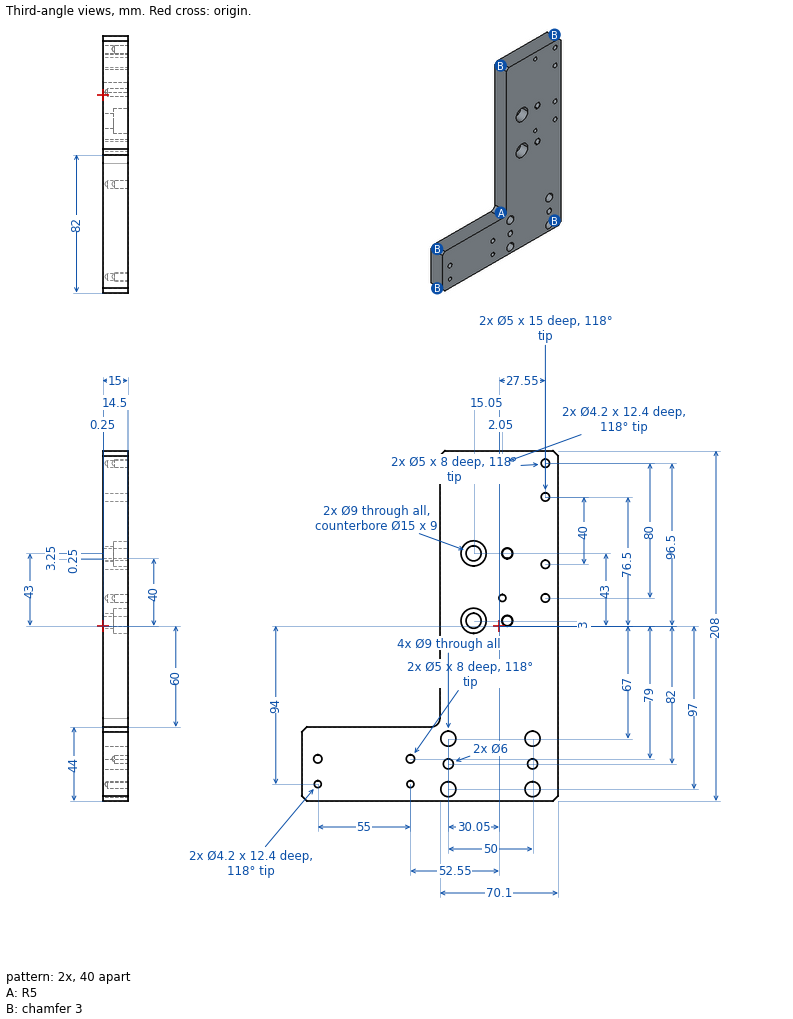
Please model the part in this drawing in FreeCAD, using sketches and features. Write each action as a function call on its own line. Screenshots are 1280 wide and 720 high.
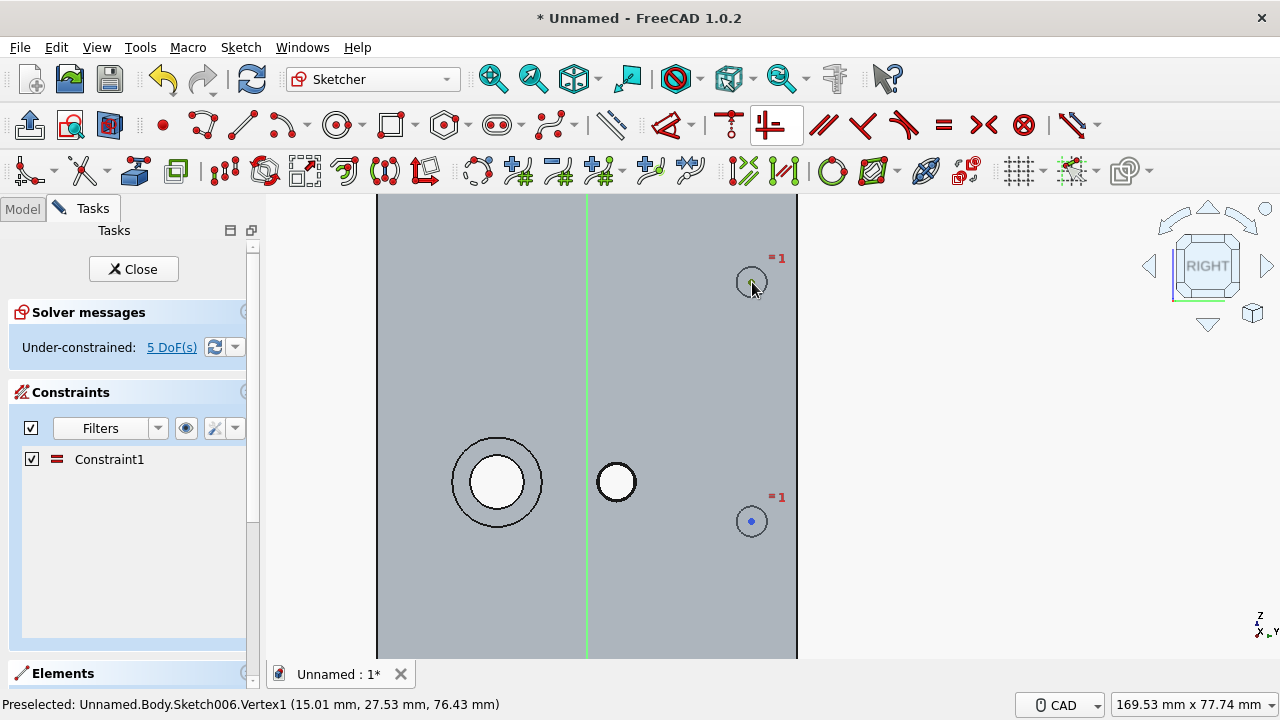
click(752, 521)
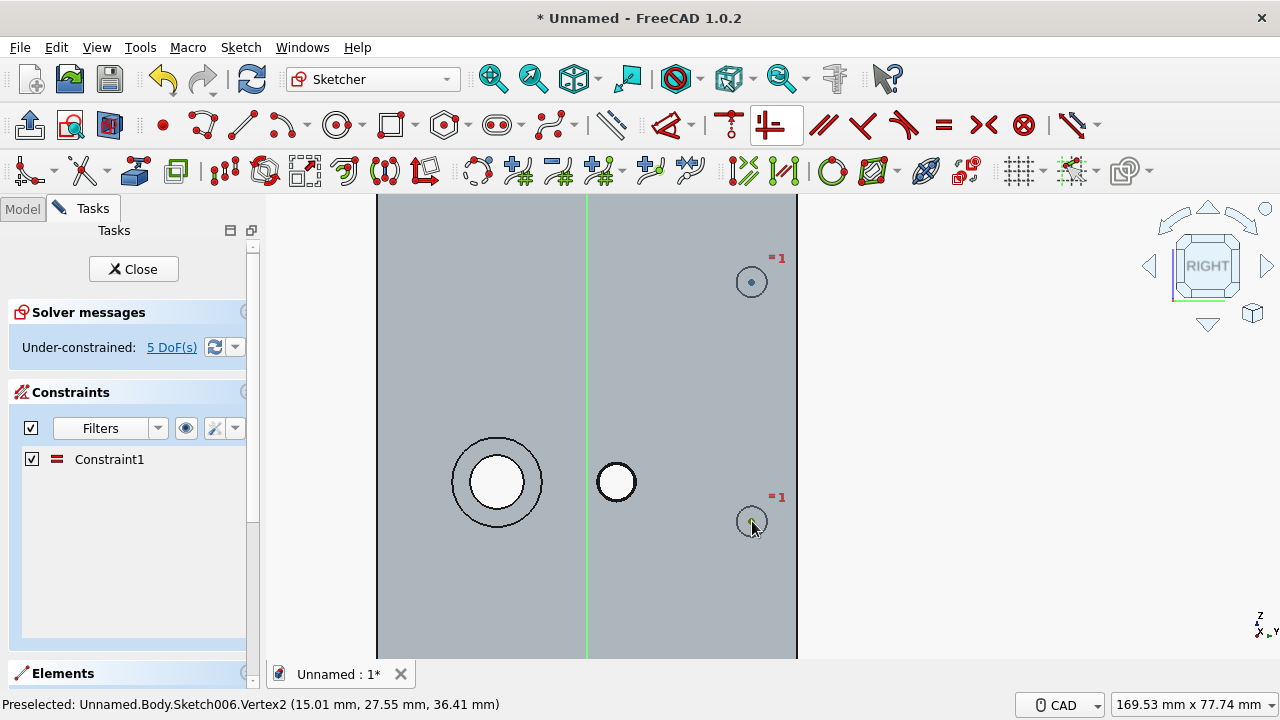
click(798, 126)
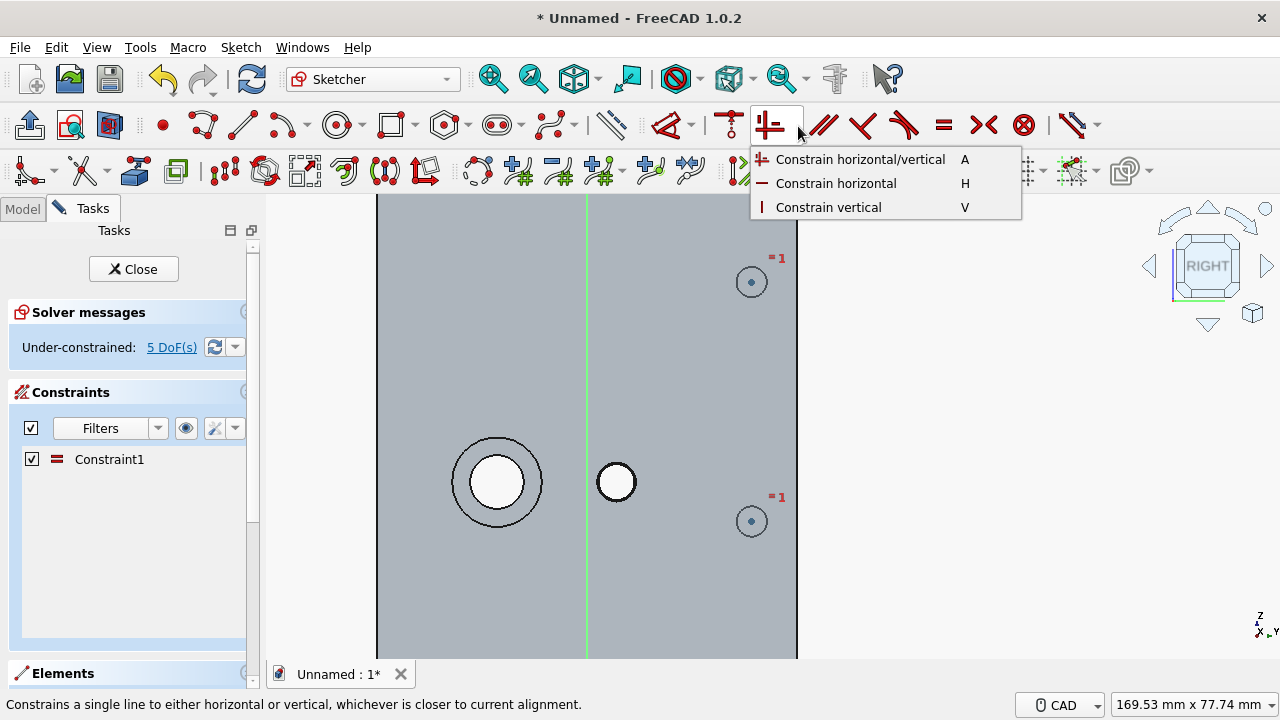
click(886, 207)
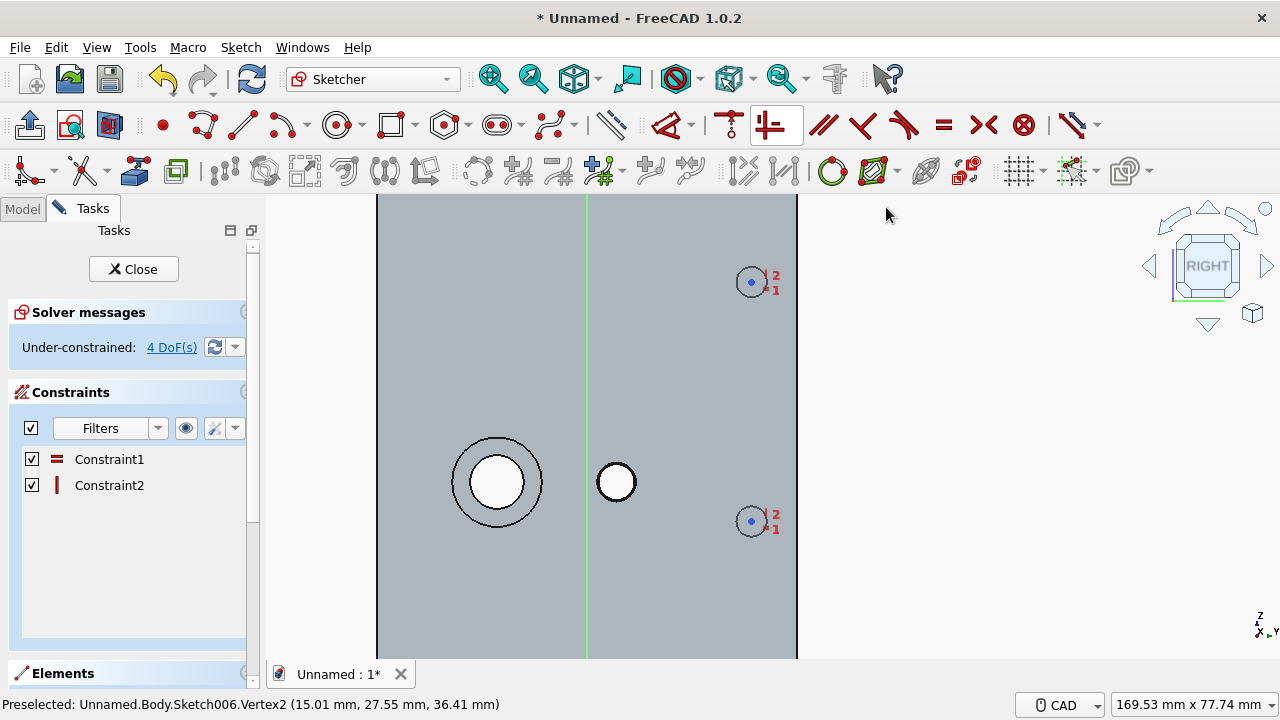
click(666, 126)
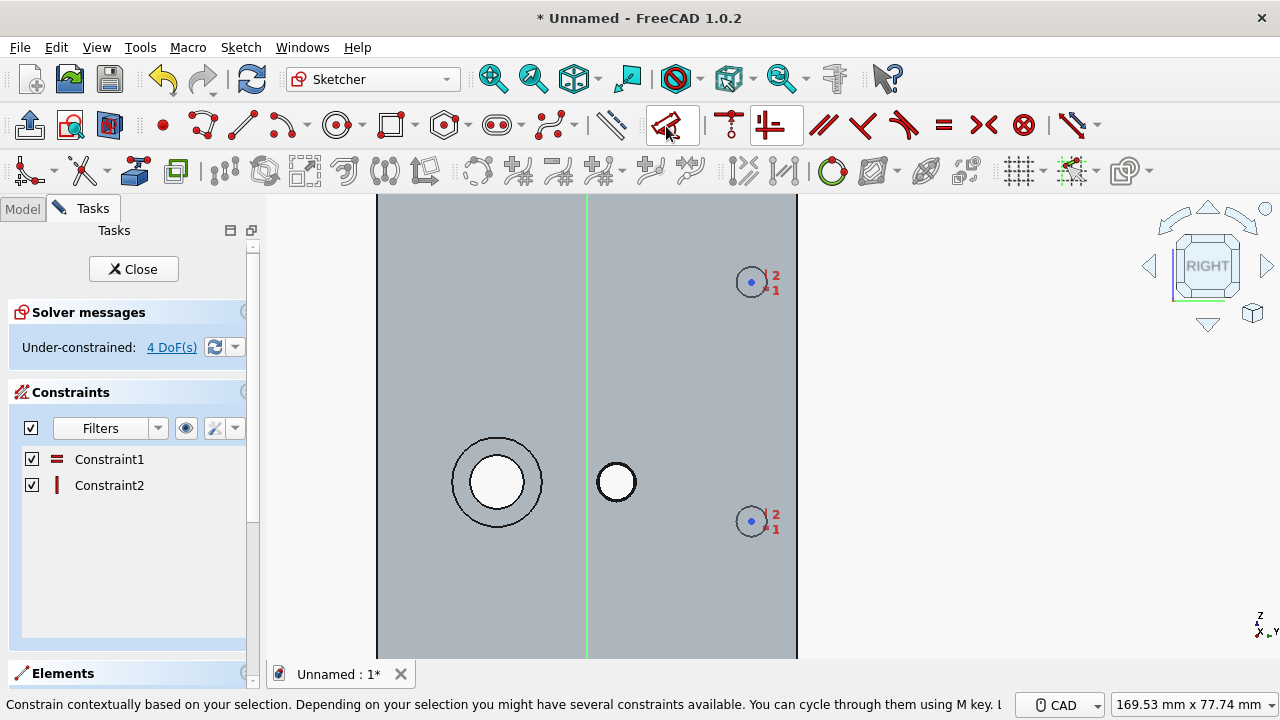
scroll(762, 271, up, 2)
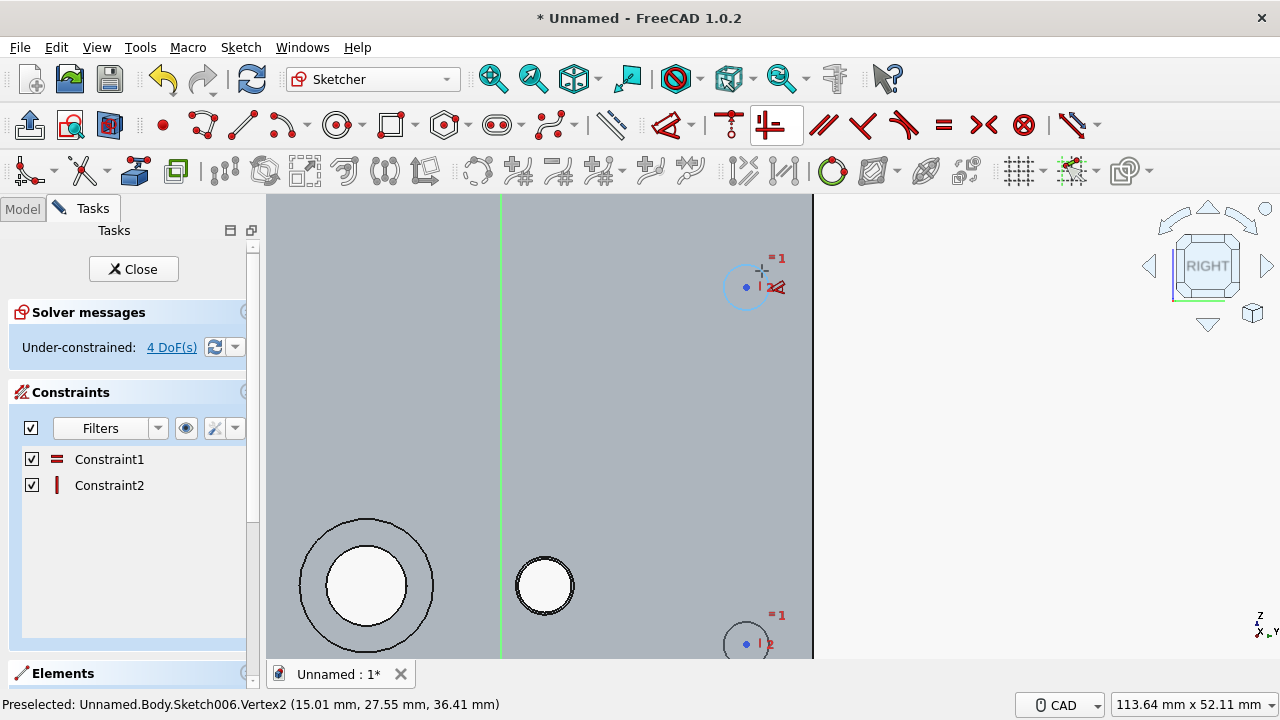
click(762, 271)
click(784, 248)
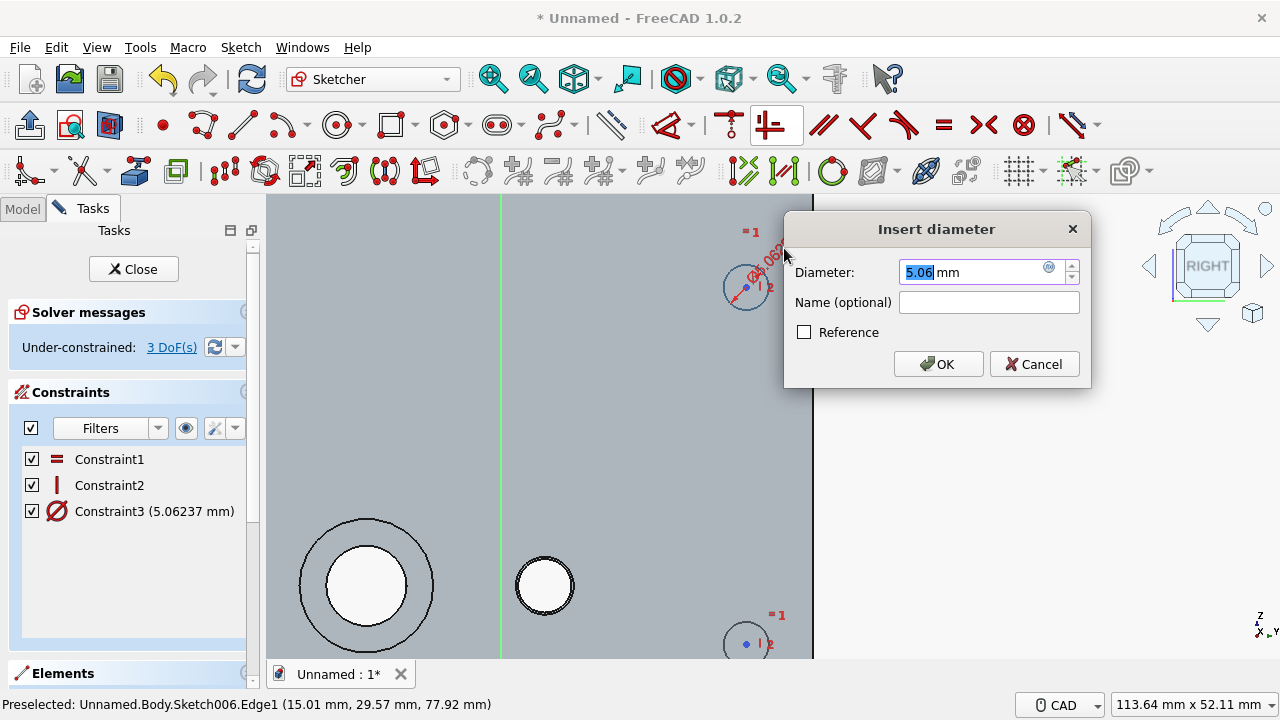
text(5)
key(Return)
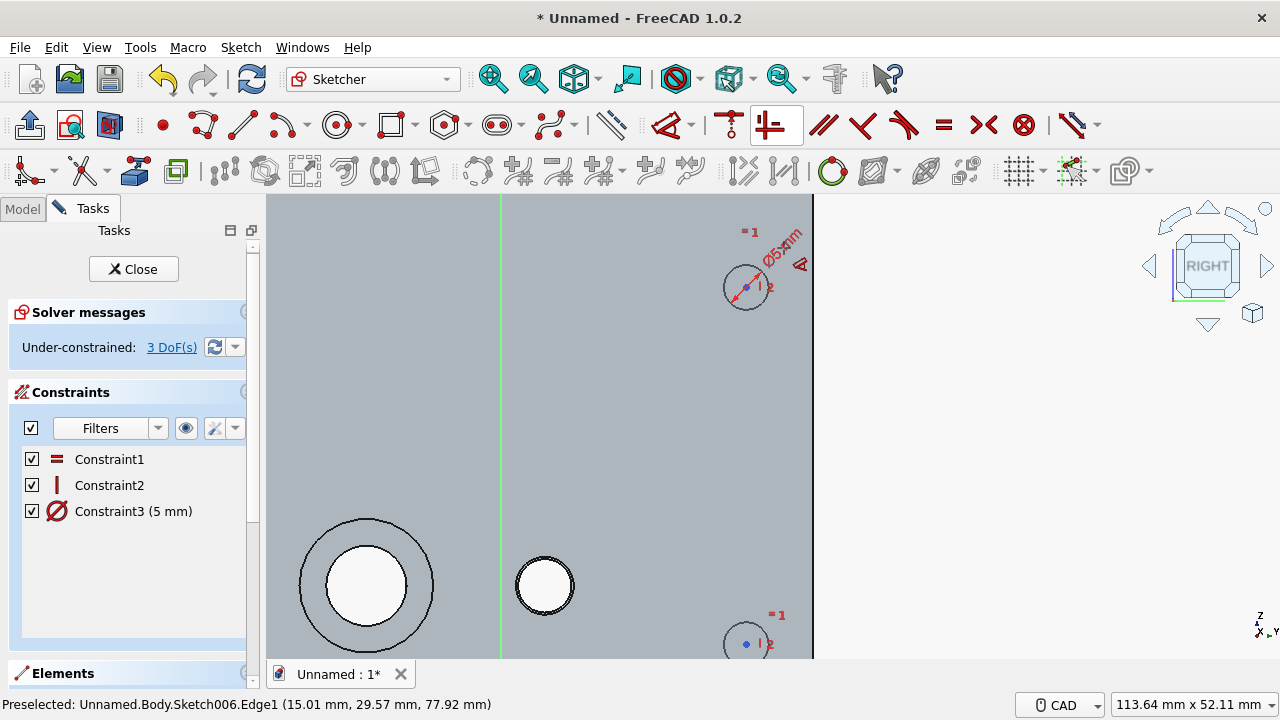
click(746, 287)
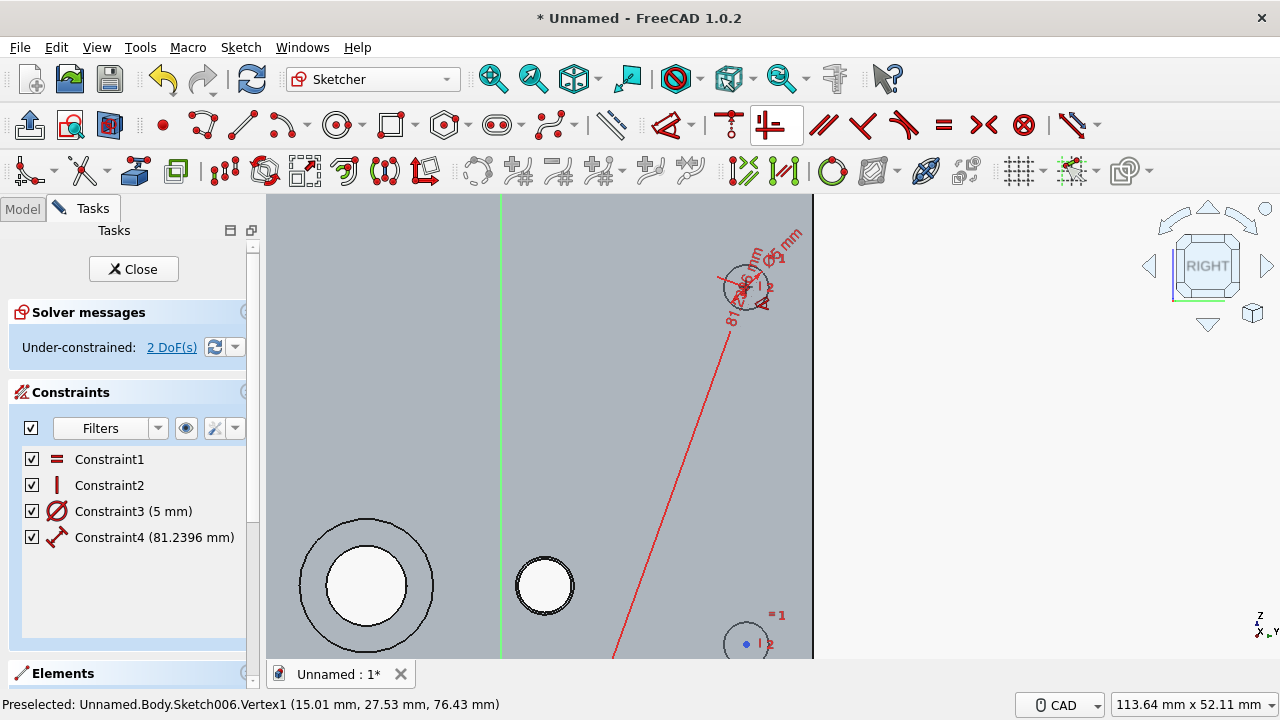
scroll(761, 271, down, 4)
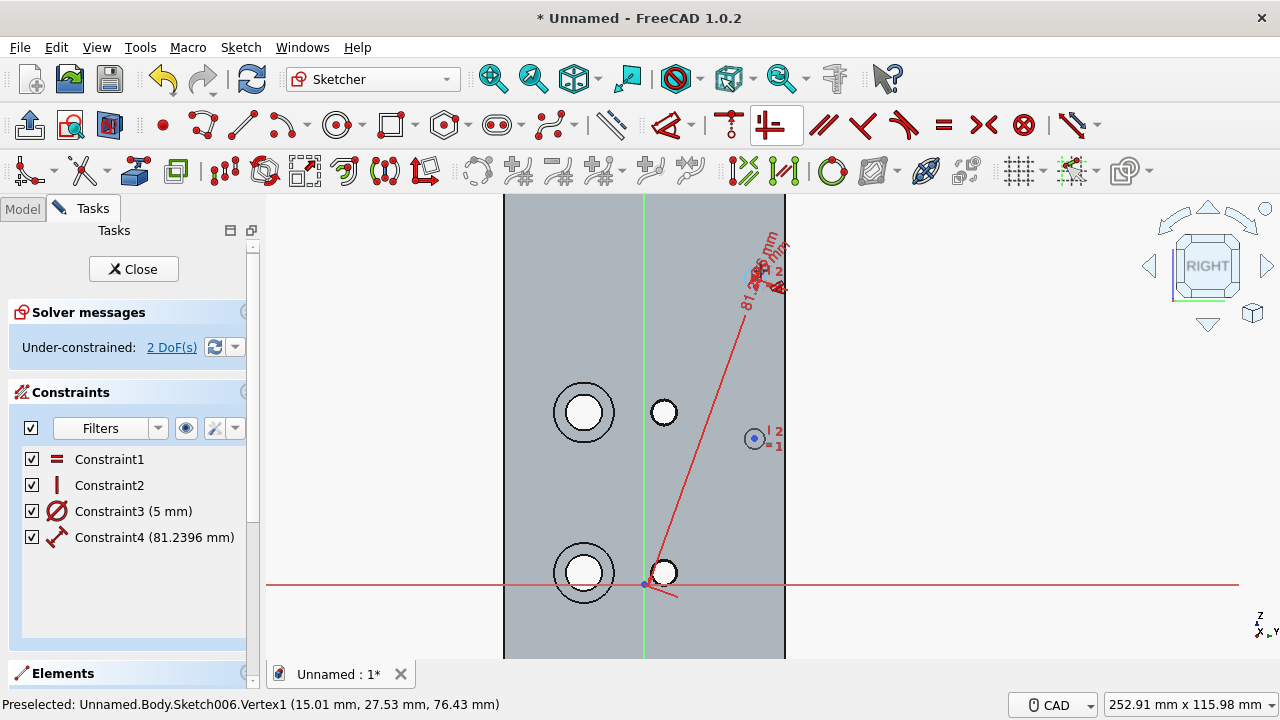
click(755, 439)
click(789, 359)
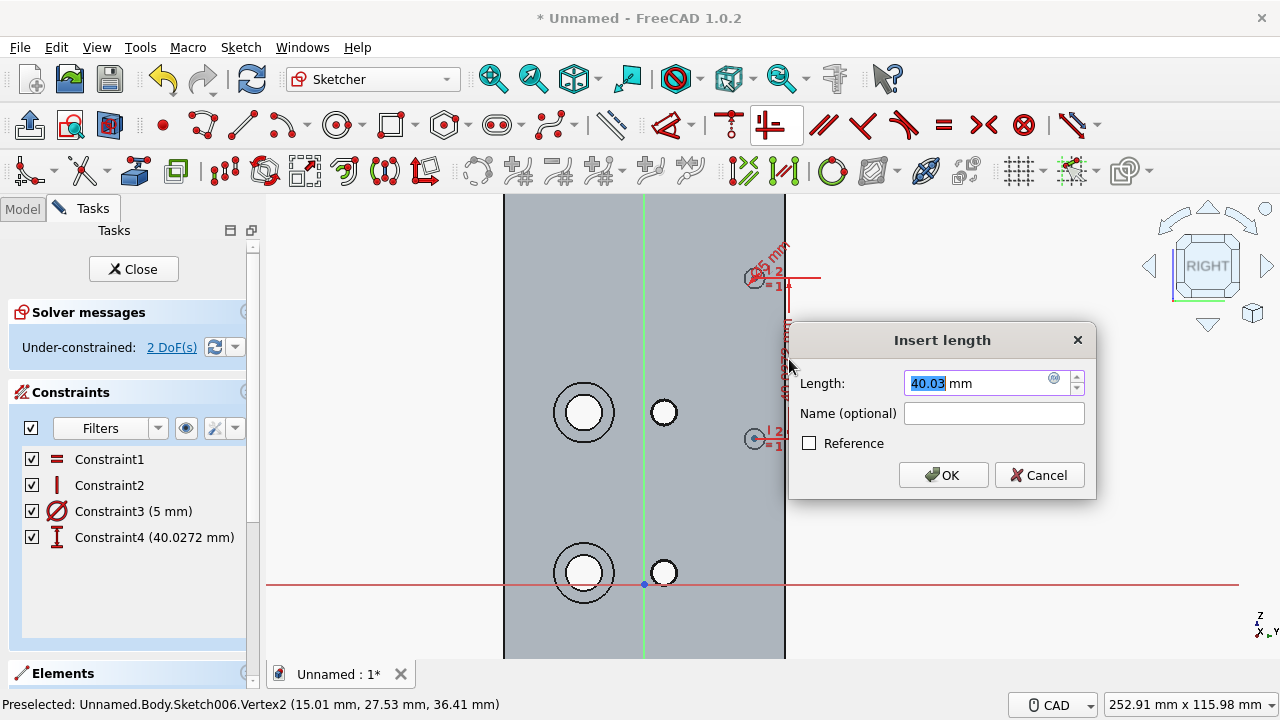
text(40)
key(Return)